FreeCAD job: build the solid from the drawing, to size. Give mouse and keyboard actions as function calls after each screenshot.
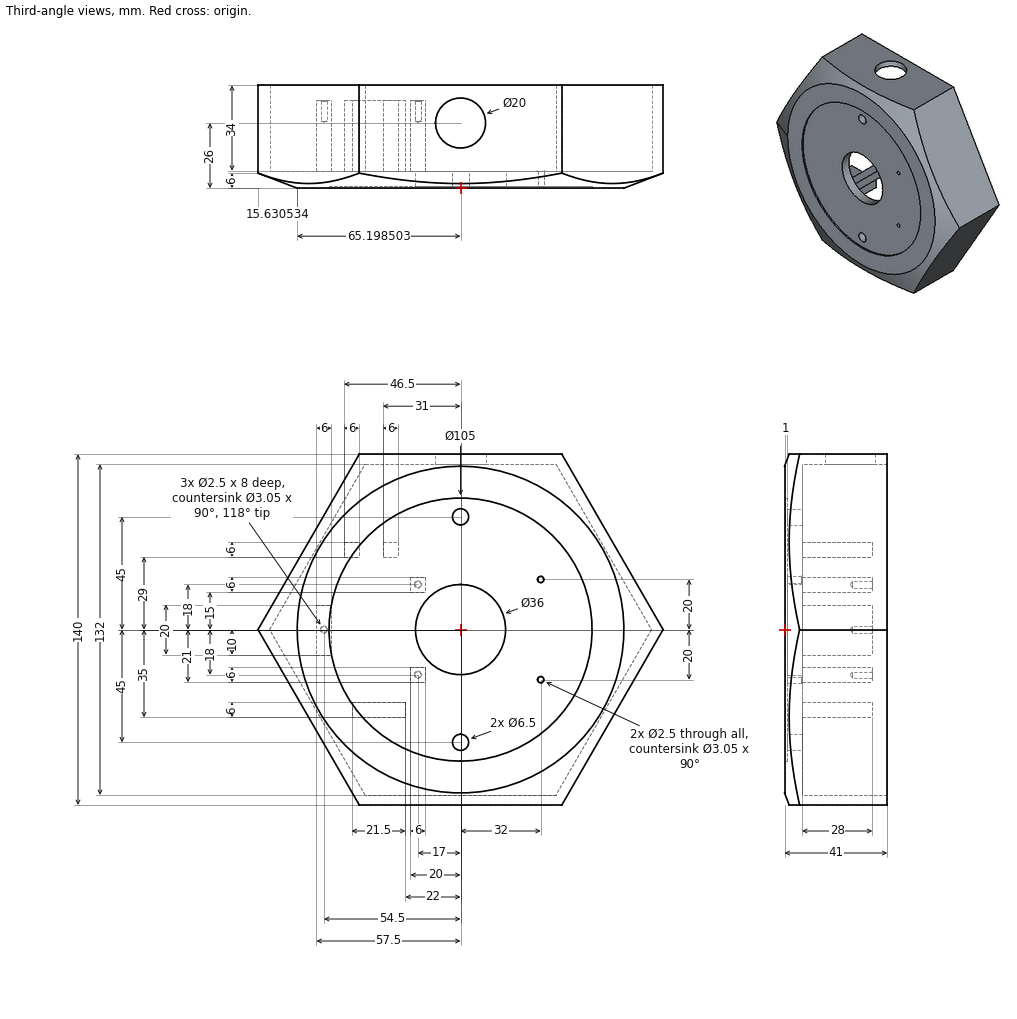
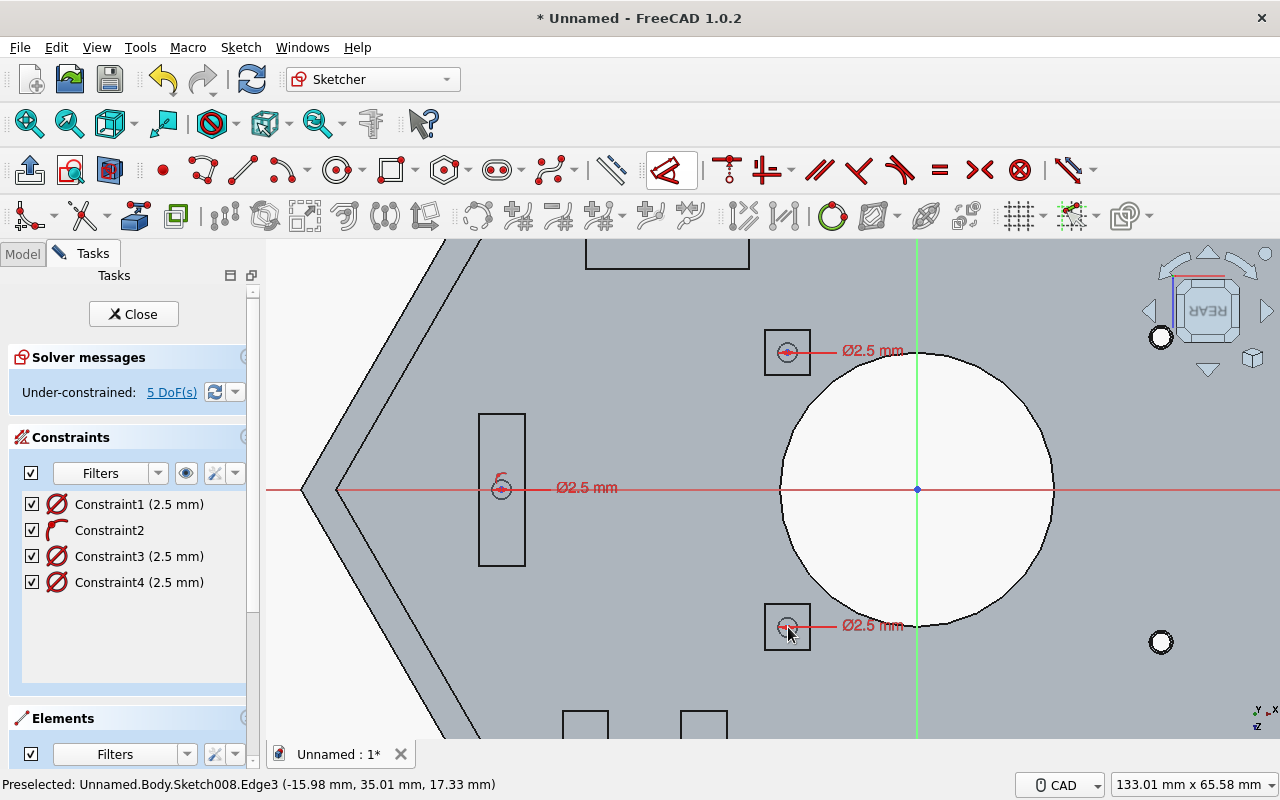
click(788, 353)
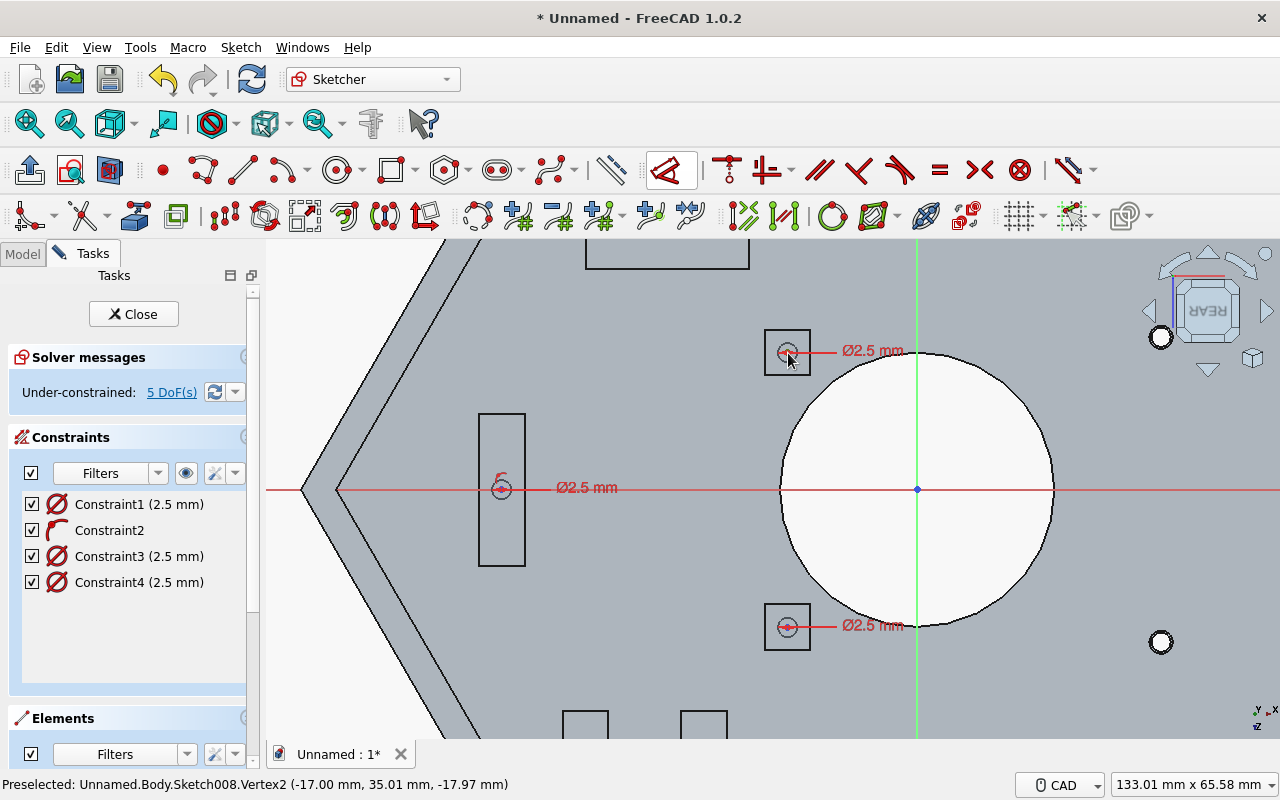
click(788, 627)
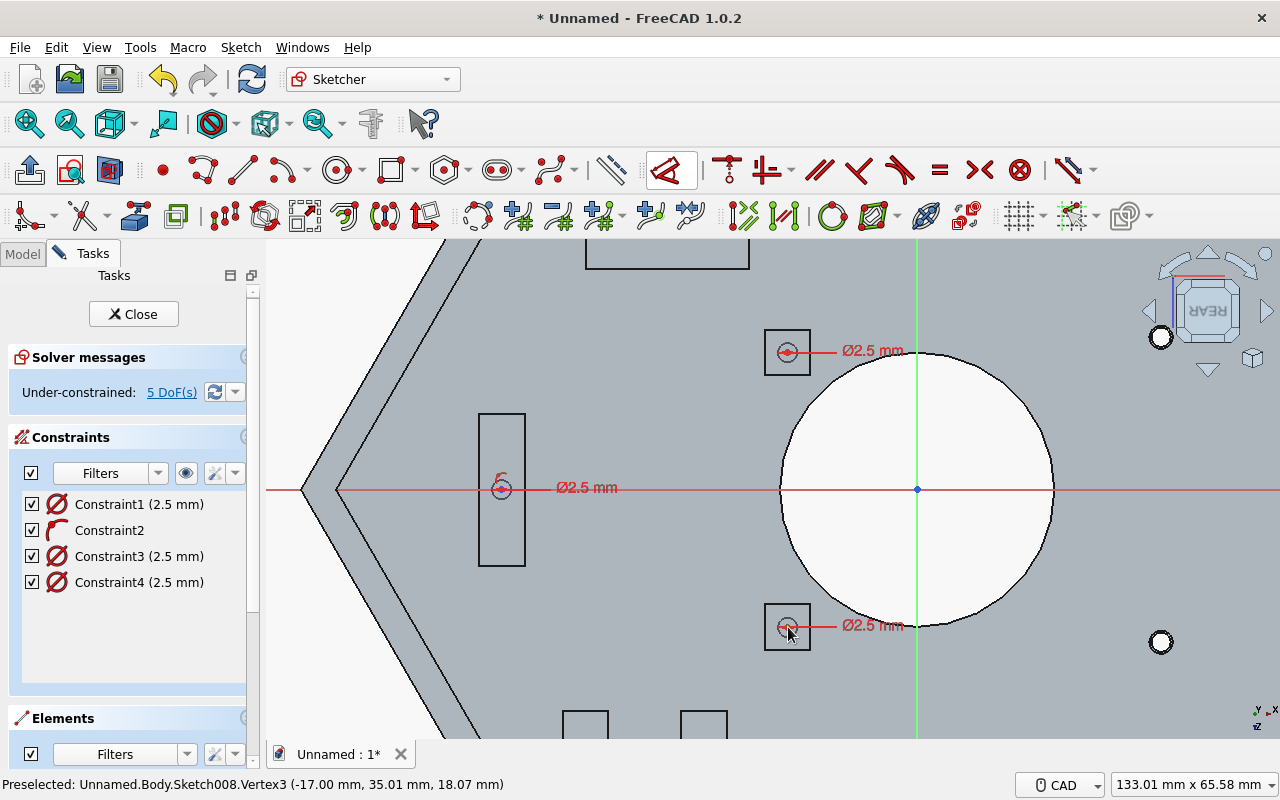
key(v)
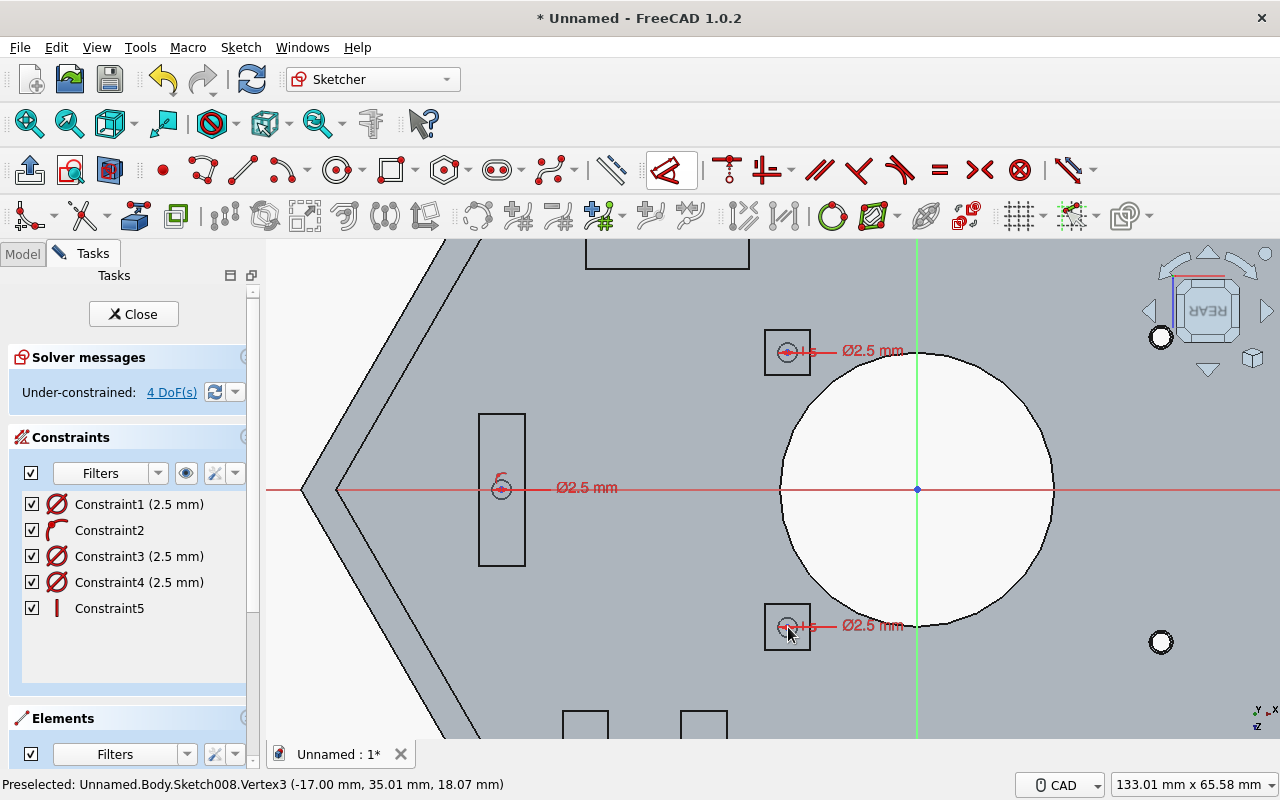
click(788, 353)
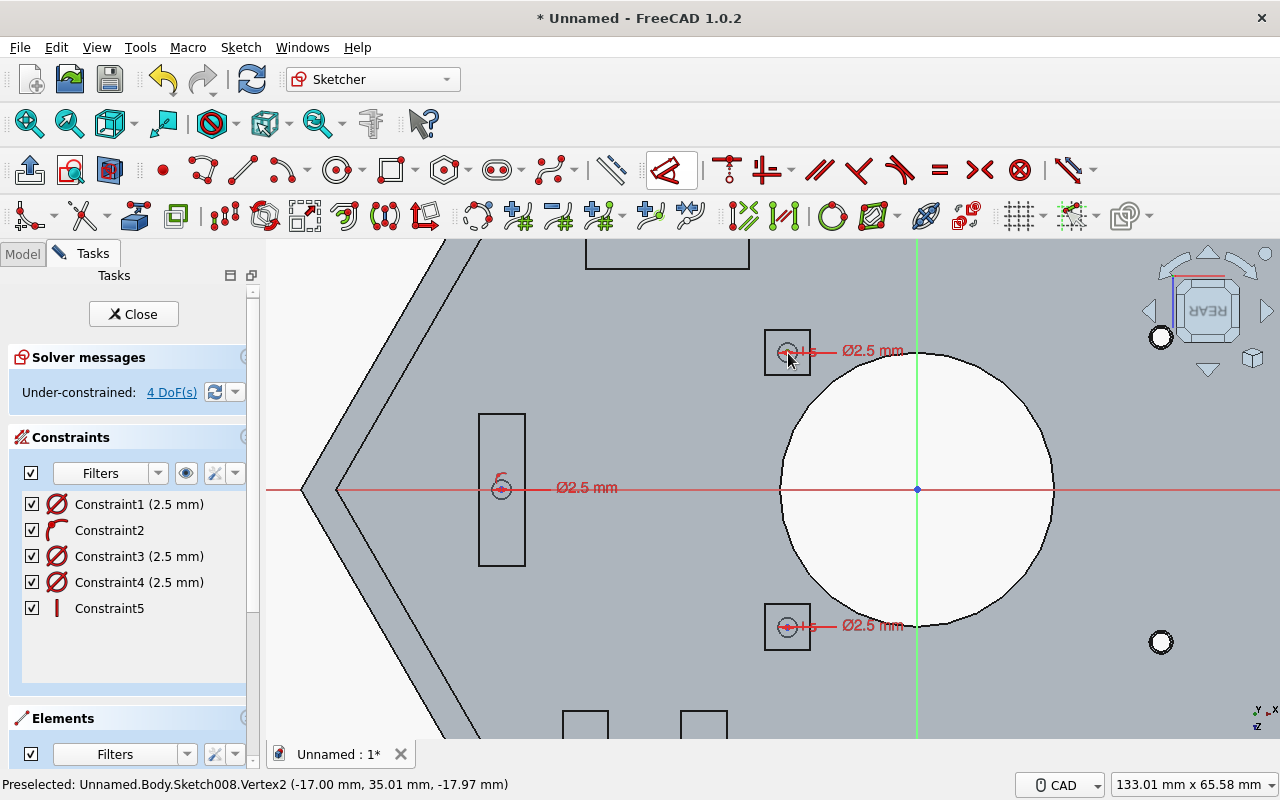
key(l)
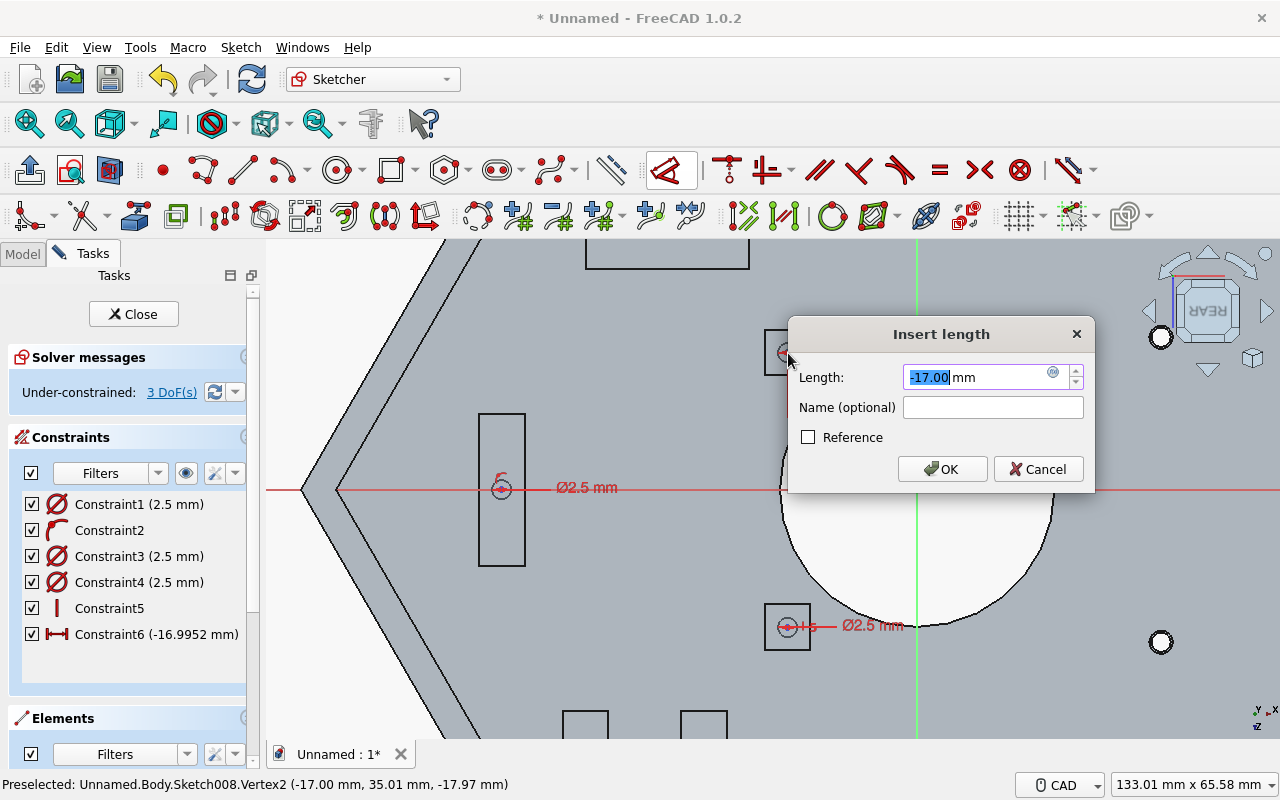
text(-17)
key(Return)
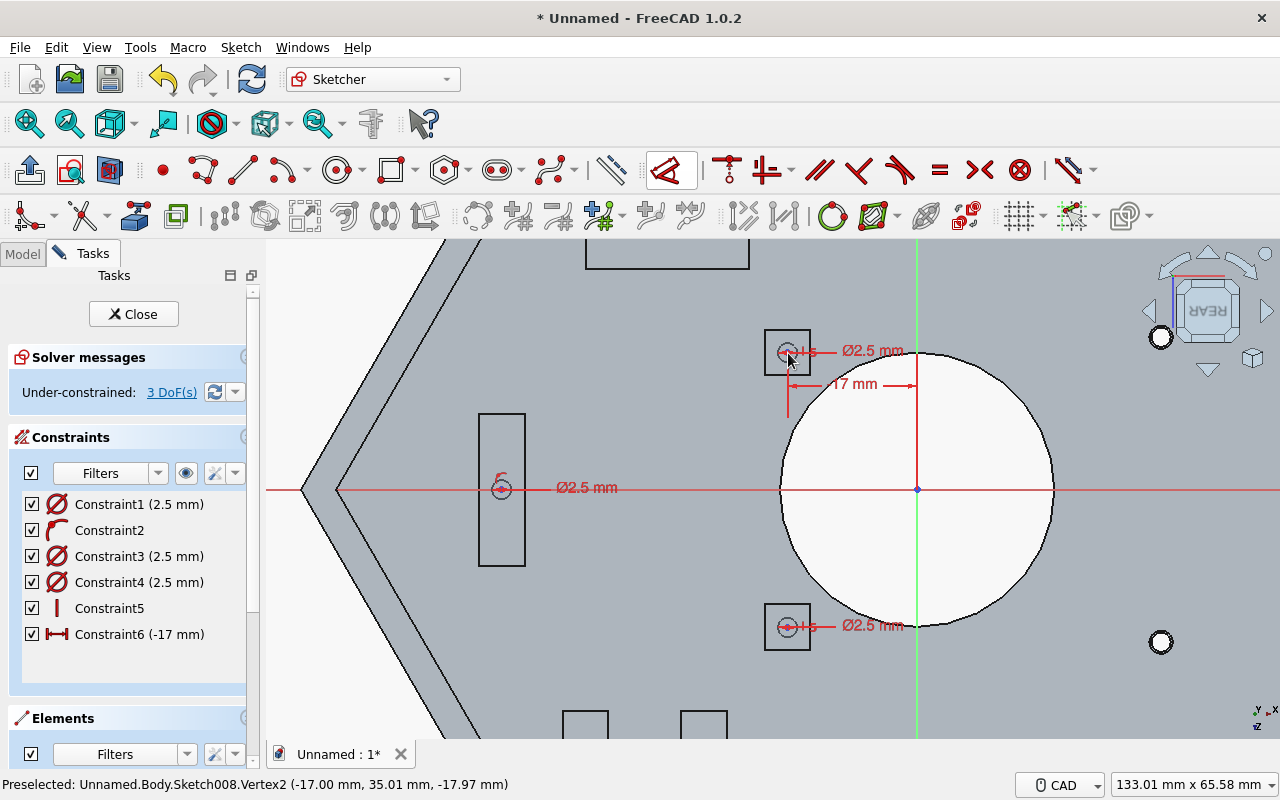
click(788, 353)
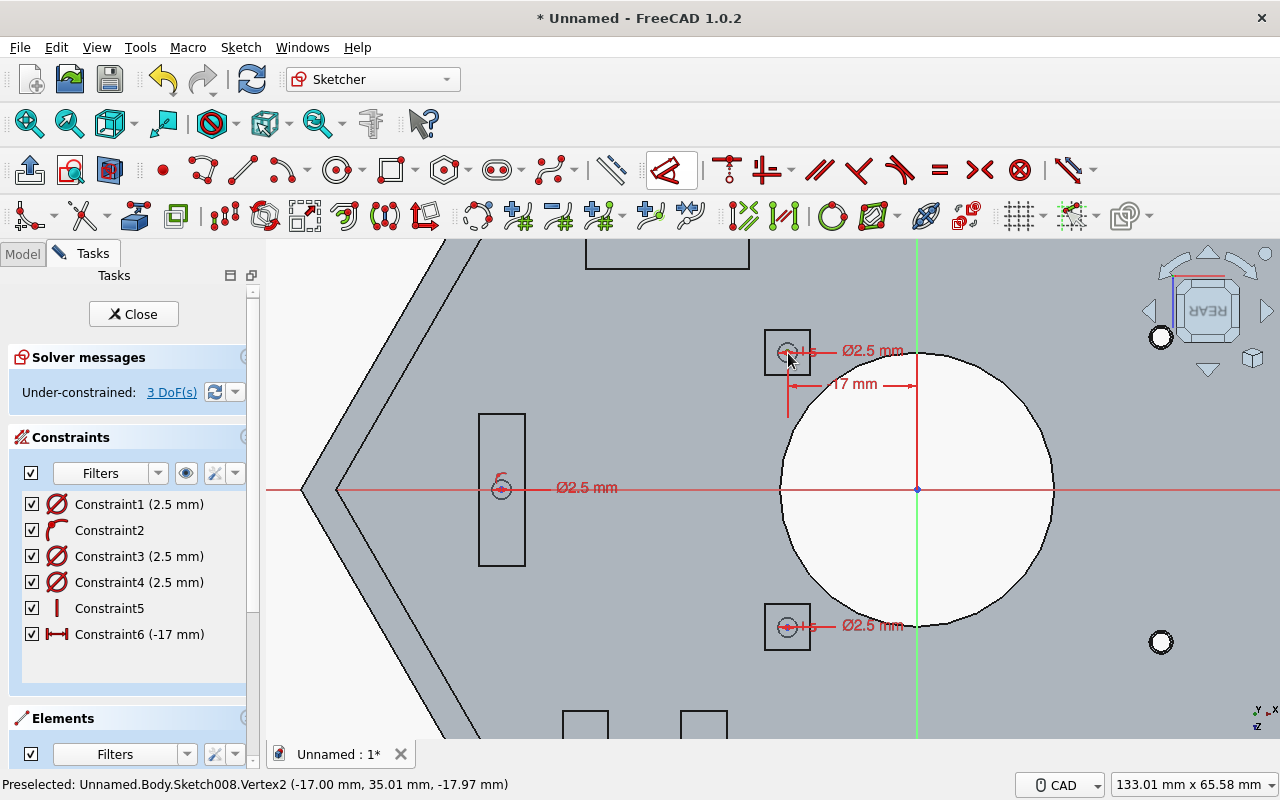
click(692, 170)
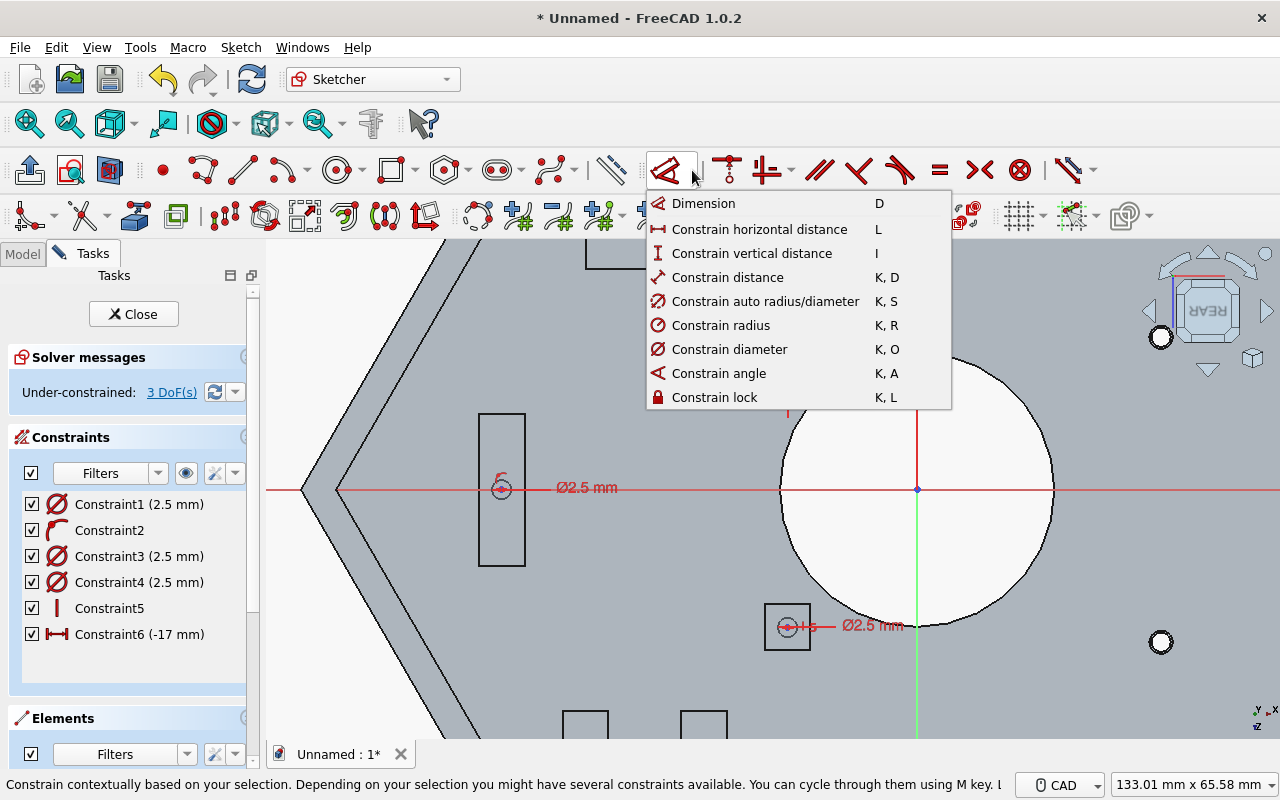
click(799, 253)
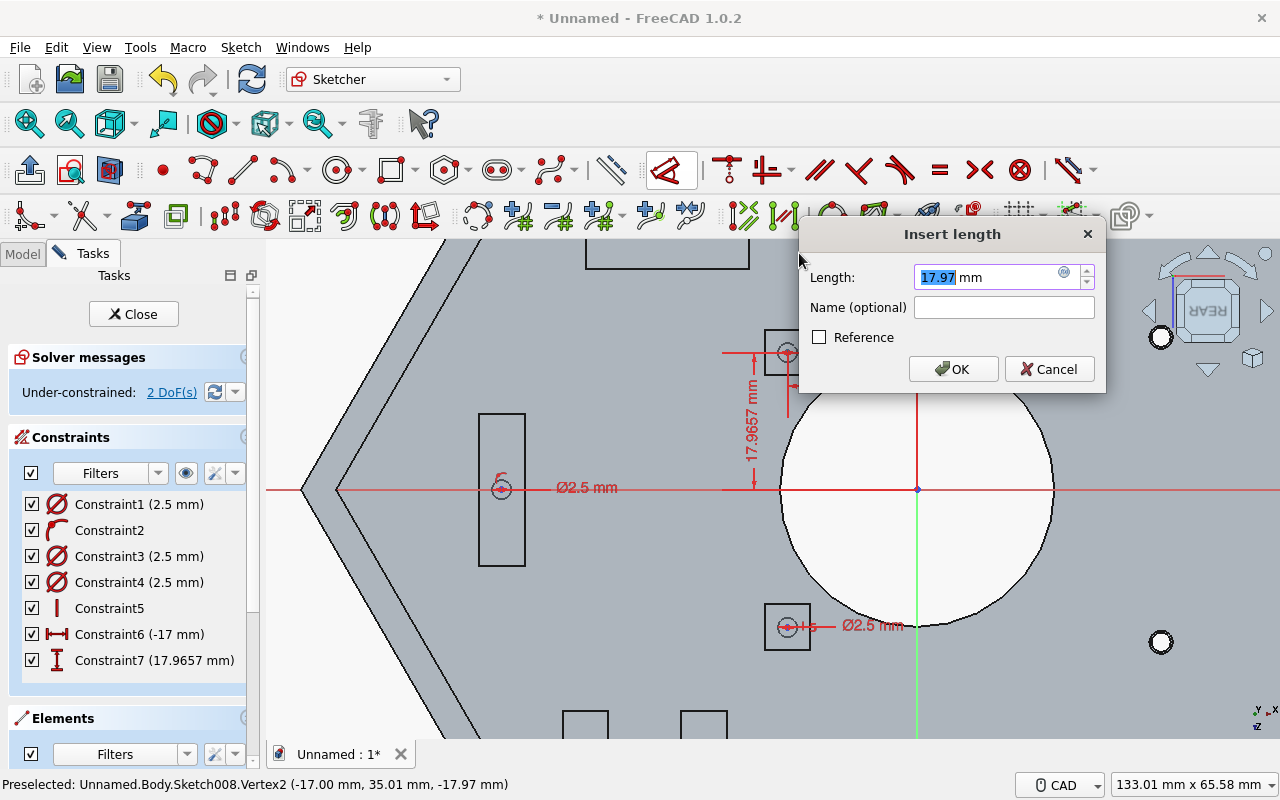
text(18)
key(Return)